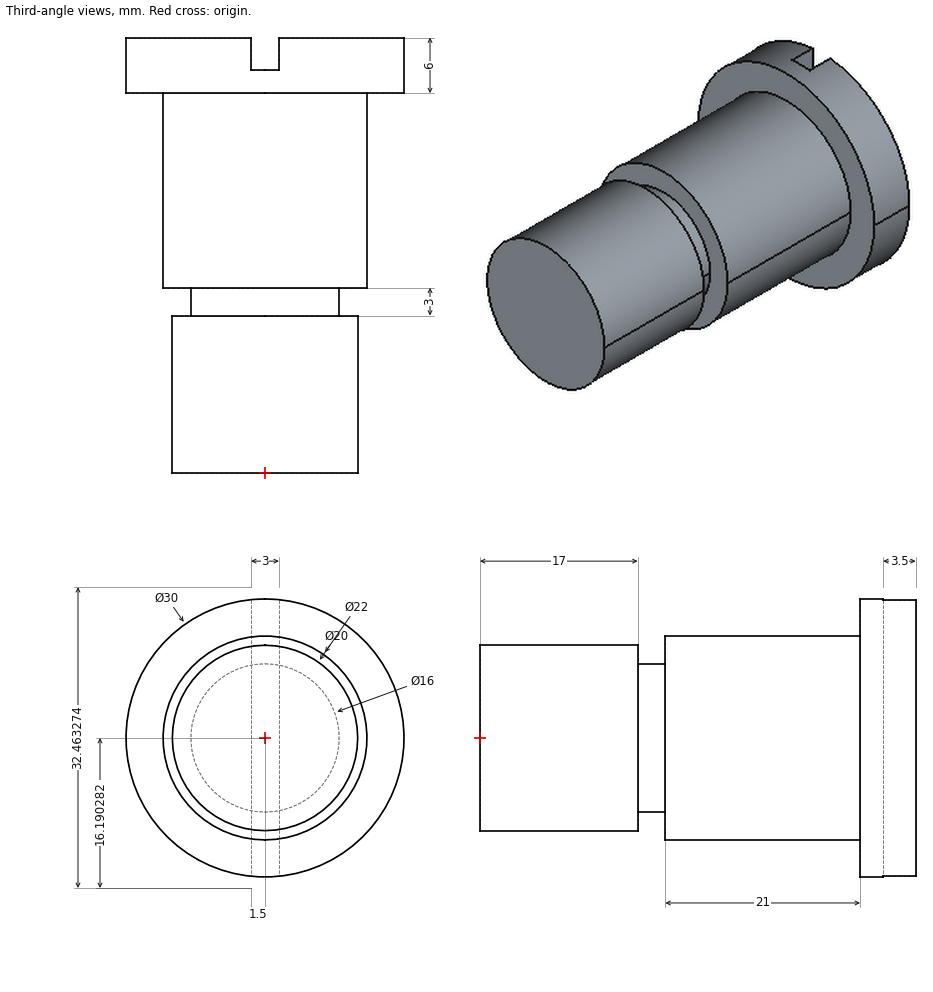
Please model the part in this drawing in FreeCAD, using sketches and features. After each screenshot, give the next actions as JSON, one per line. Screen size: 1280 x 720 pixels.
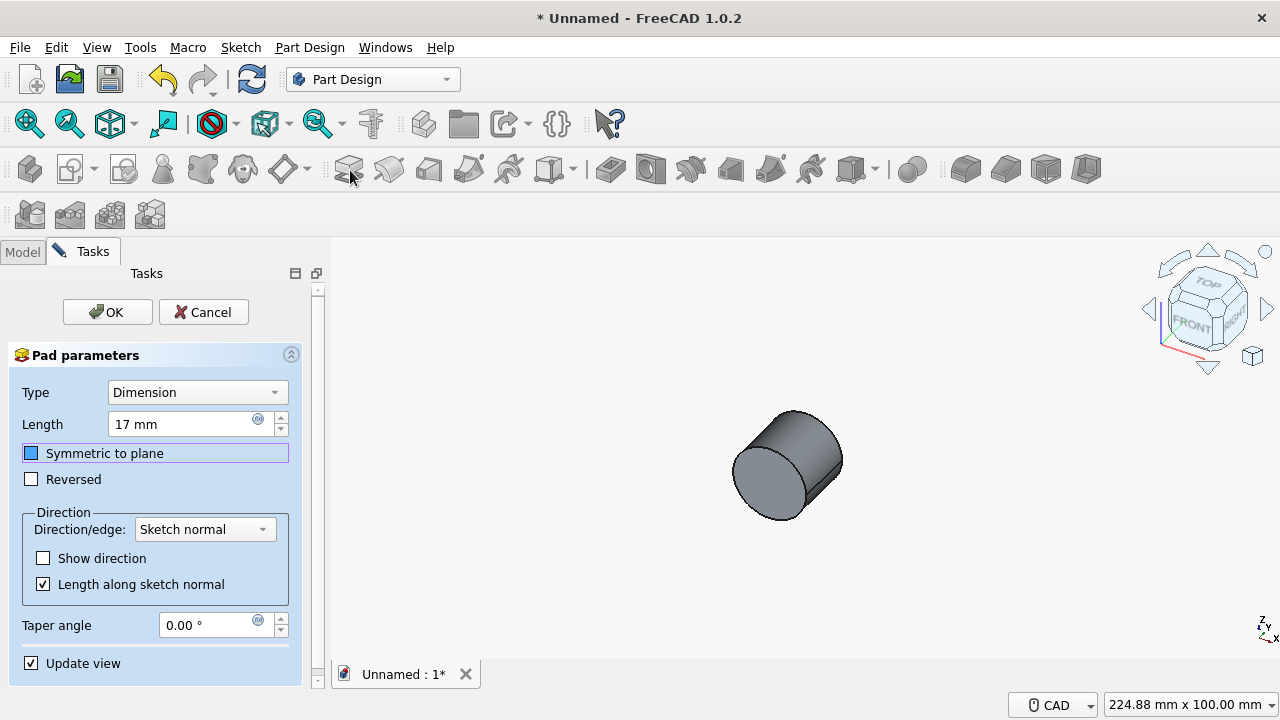
{"action": "left_click", "coordinate": [30, 479]}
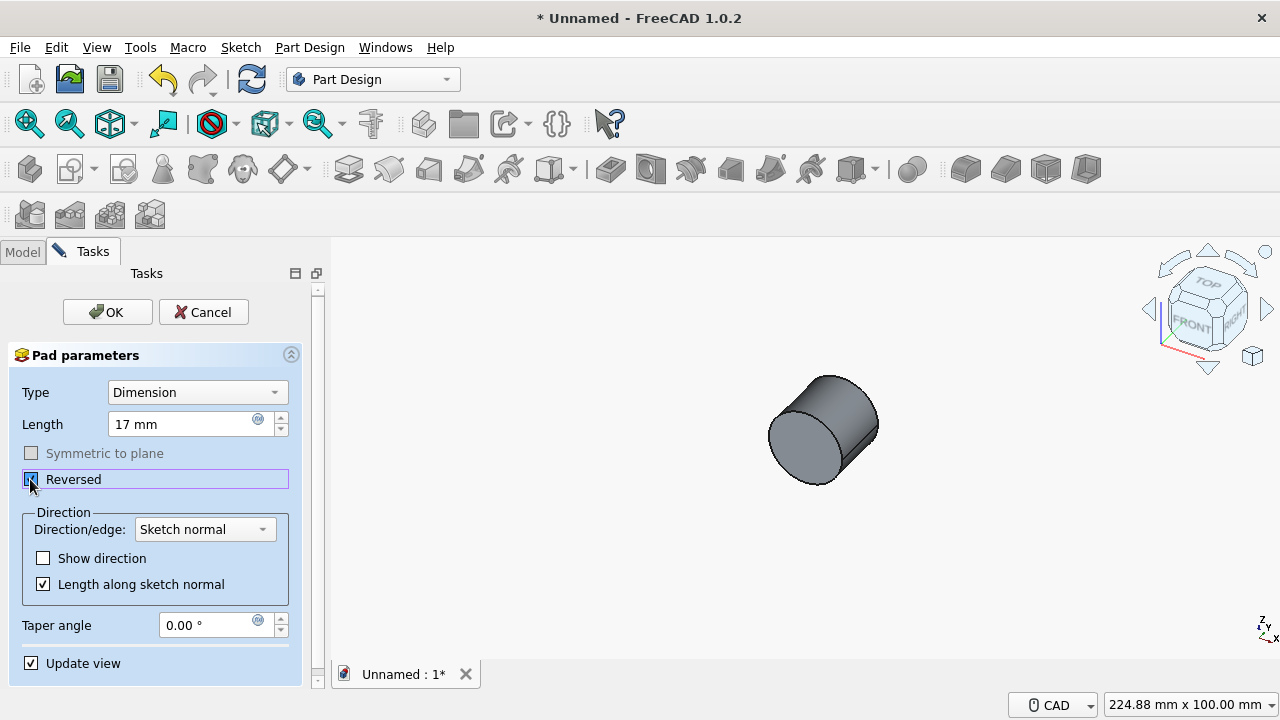
{"action": "left_click", "coordinate": [108, 312]}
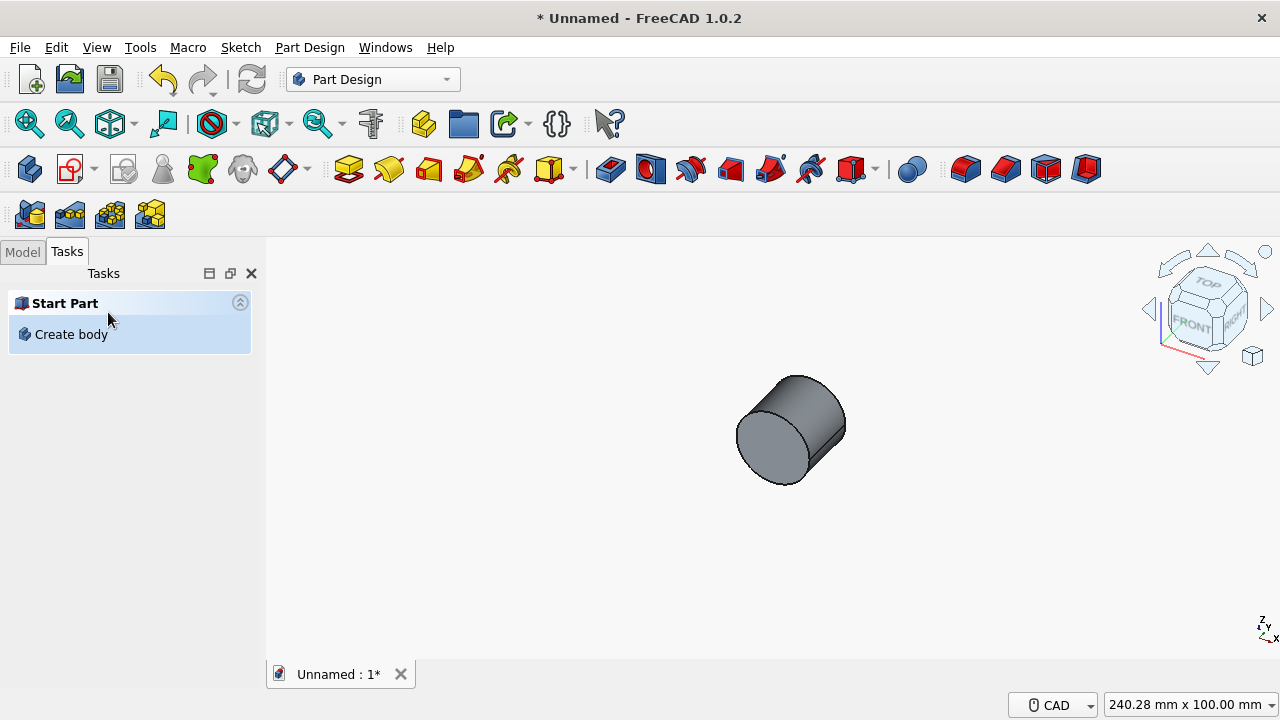
{"action": "left_click", "coordinate": [30, 124]}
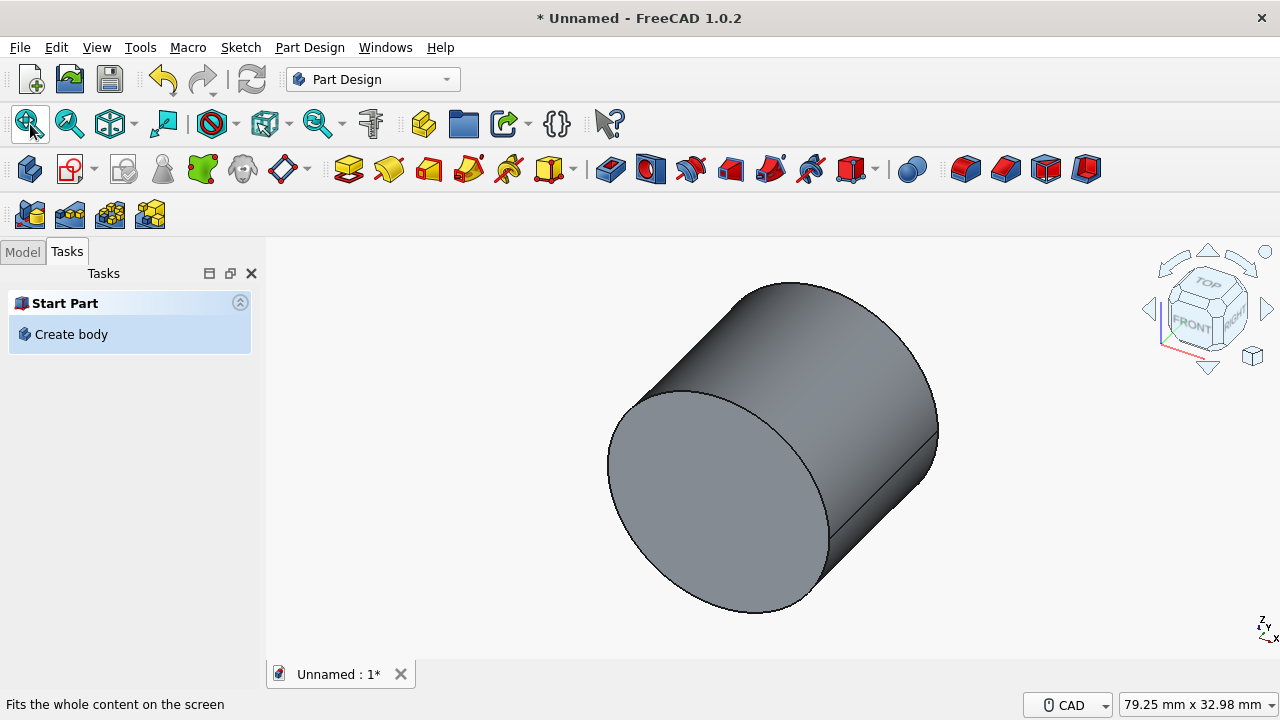
{"action": "key", "text": "4"}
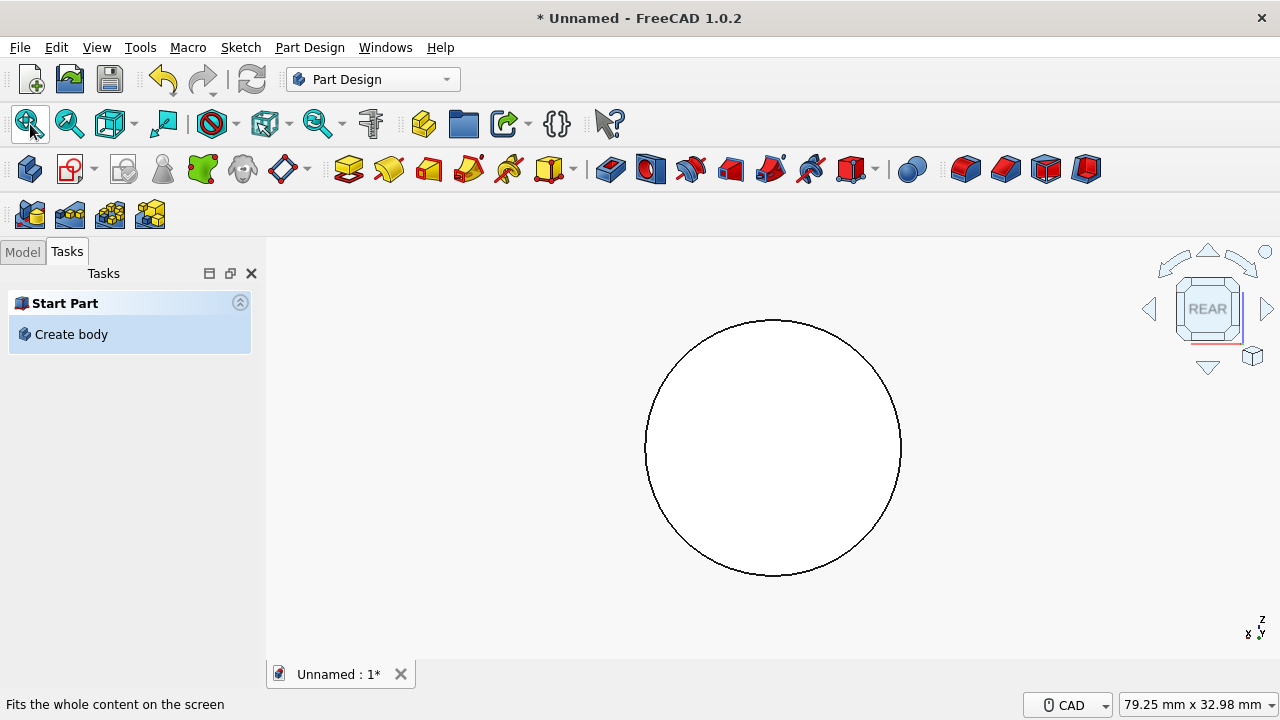
{"action": "left_click", "coordinate": [773, 447]}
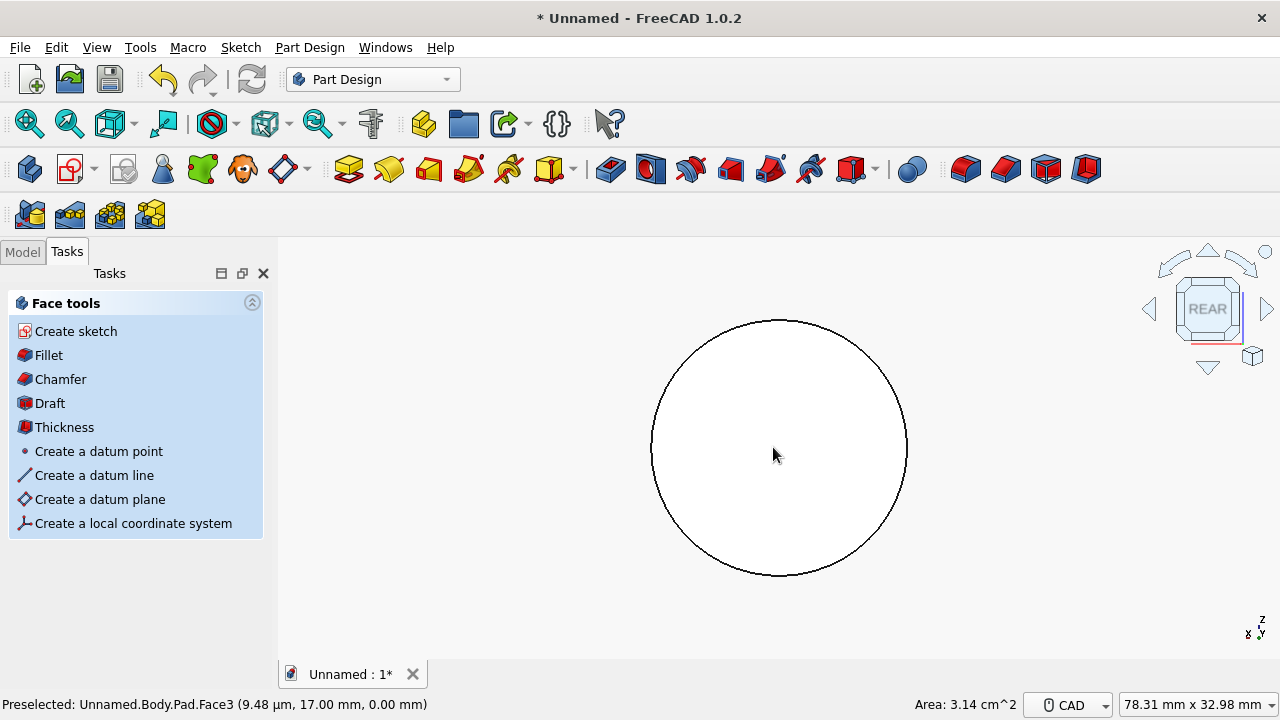
{"action": "left_click", "coordinate": [70, 170]}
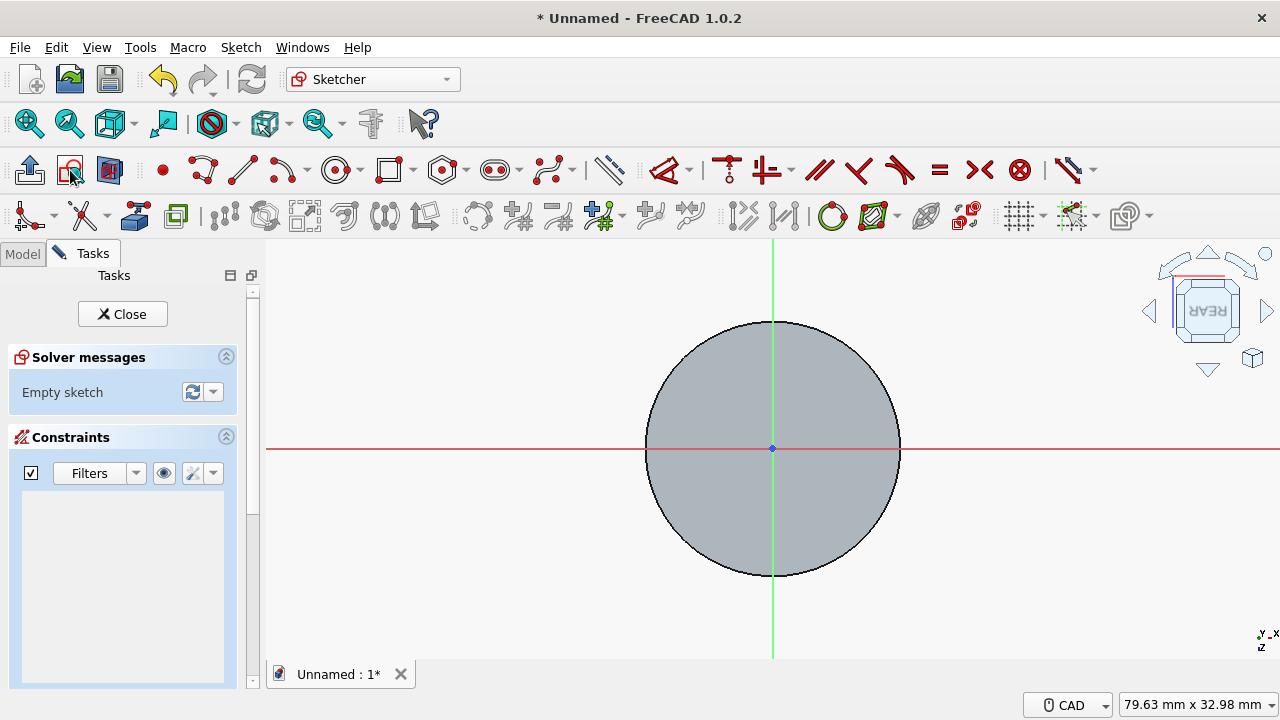
{"action": "left_click", "coordinate": [336, 170]}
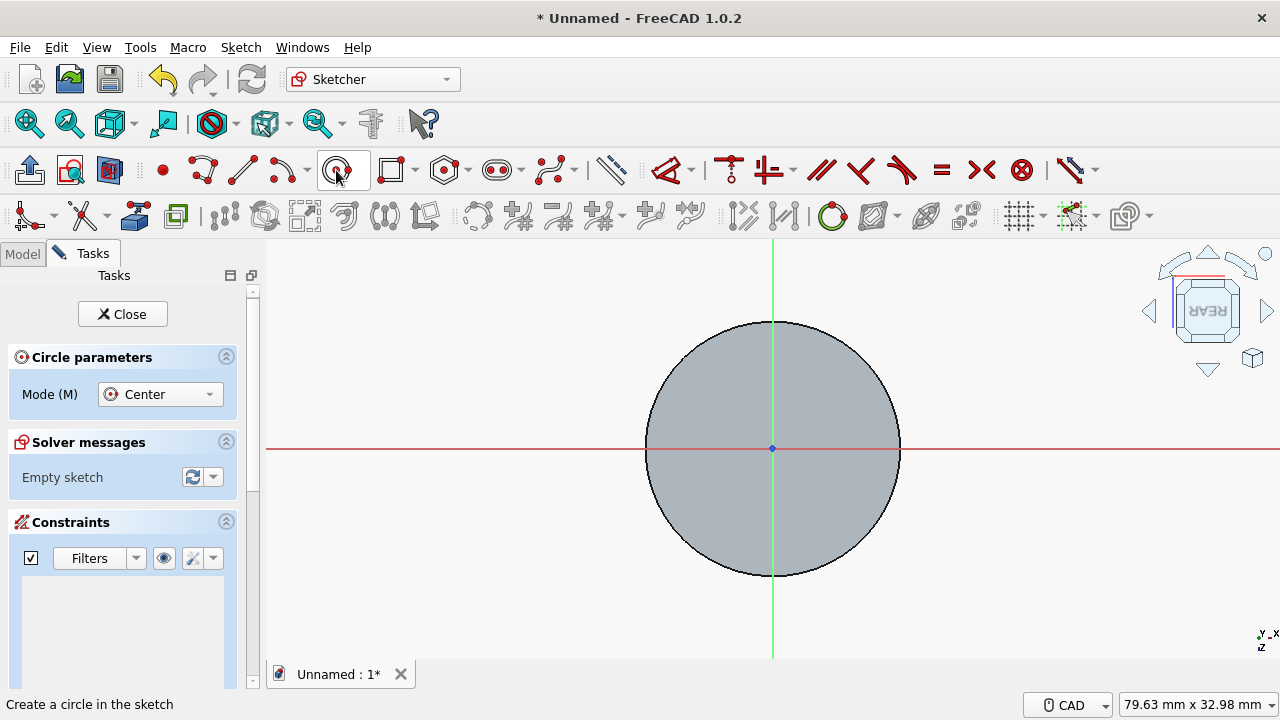
{"action": "left_click", "coordinate": [773, 449]}
{"action": "mouse_move", "coordinate": [845, 377]}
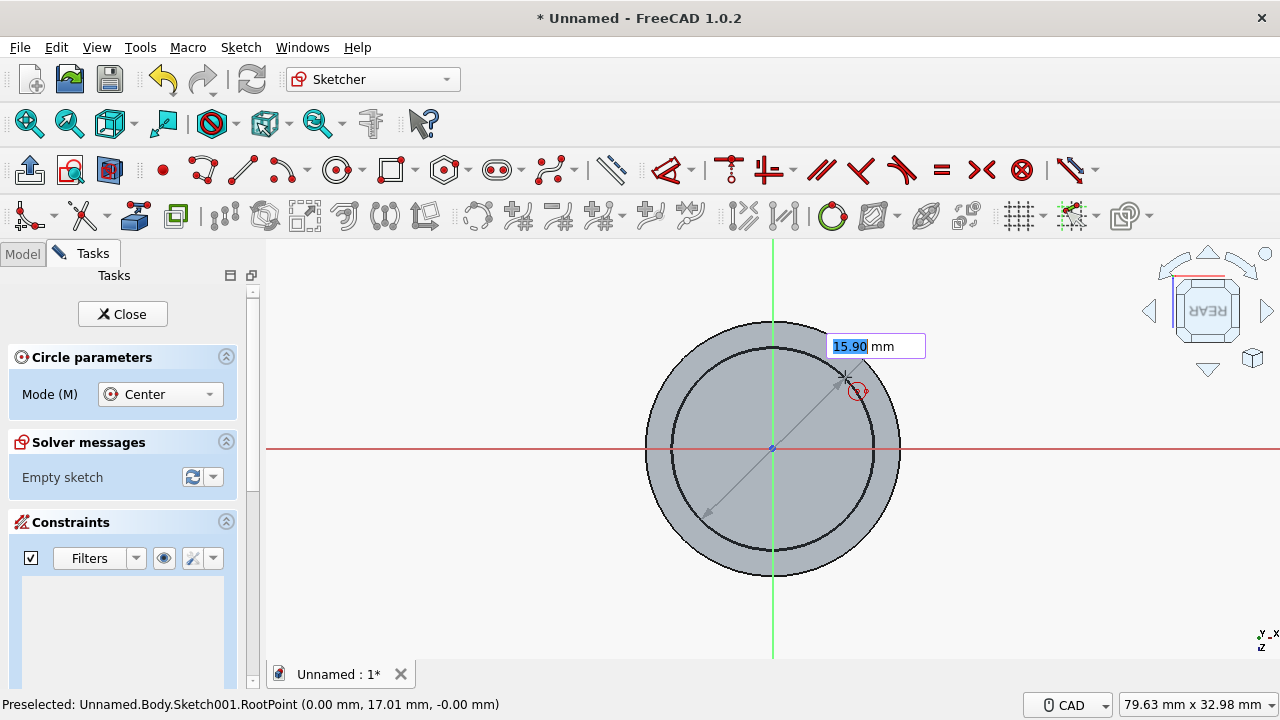
{"action": "type", "text": "16"}
{"action": "key", "text": "Return"}
{"action": "key", "text": "Escape"}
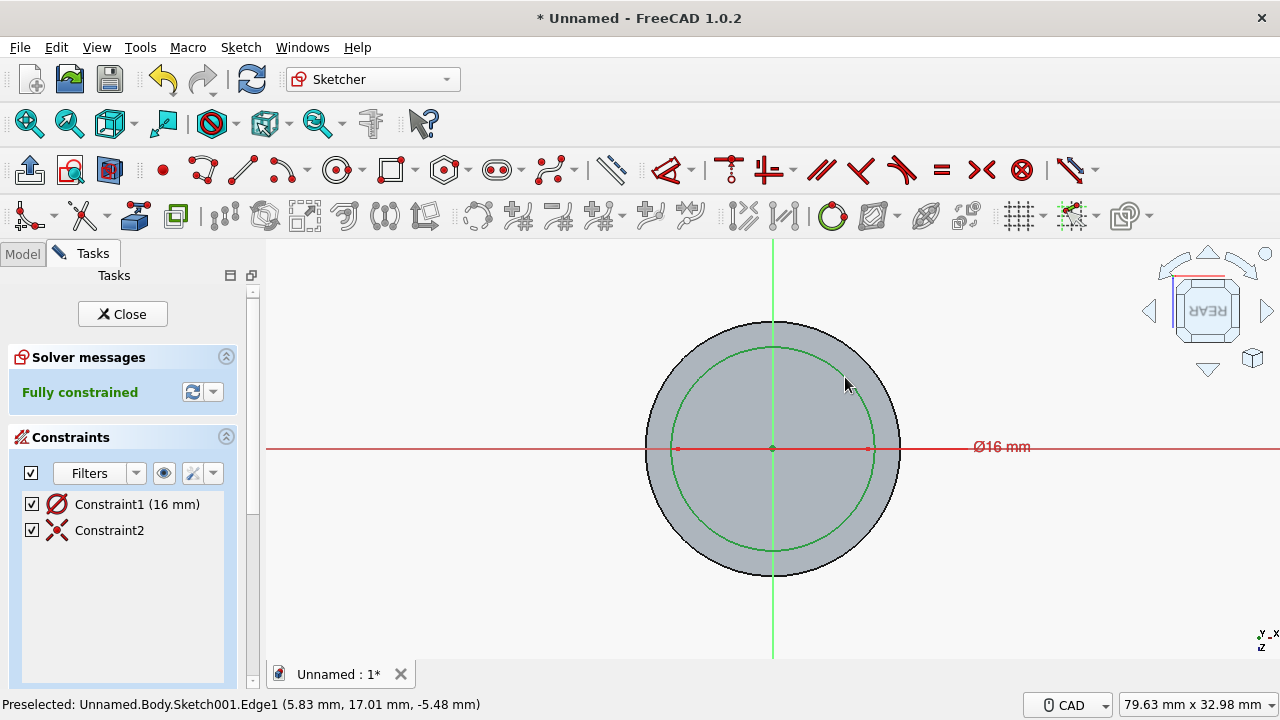
{"action": "left_click", "coordinate": [123, 314]}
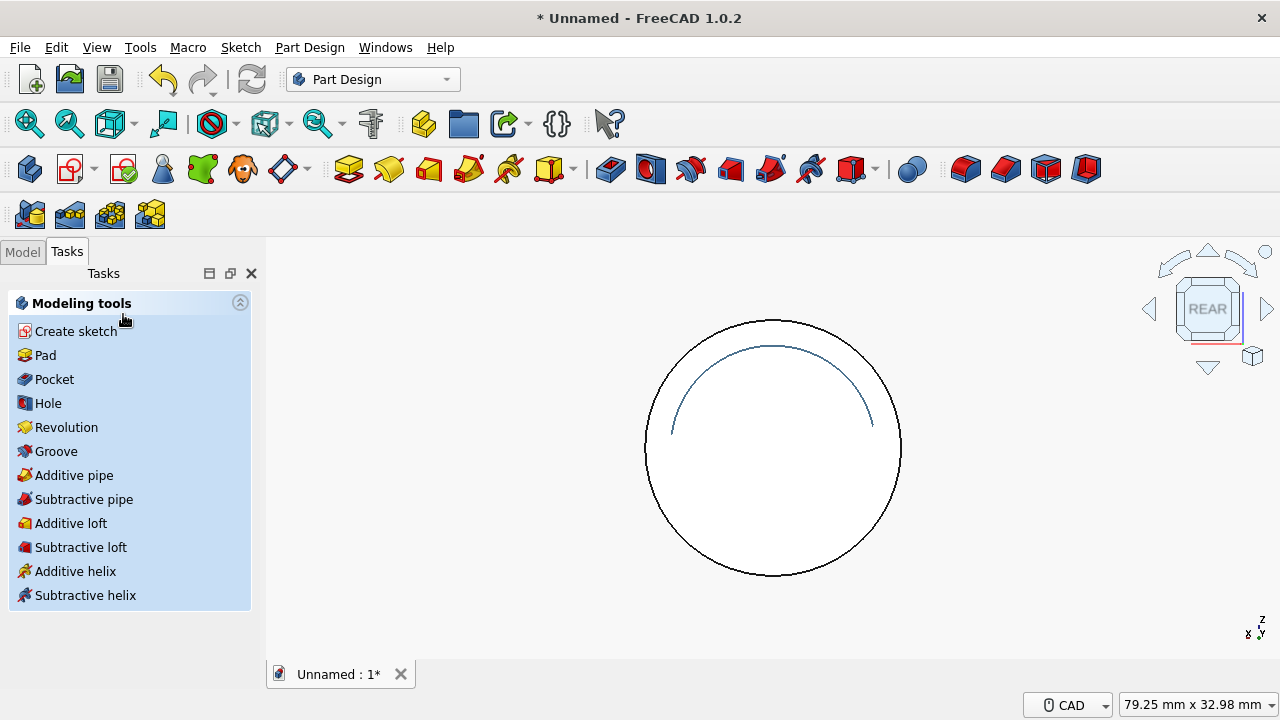
{"action": "left_click", "coordinate": [350, 170]}